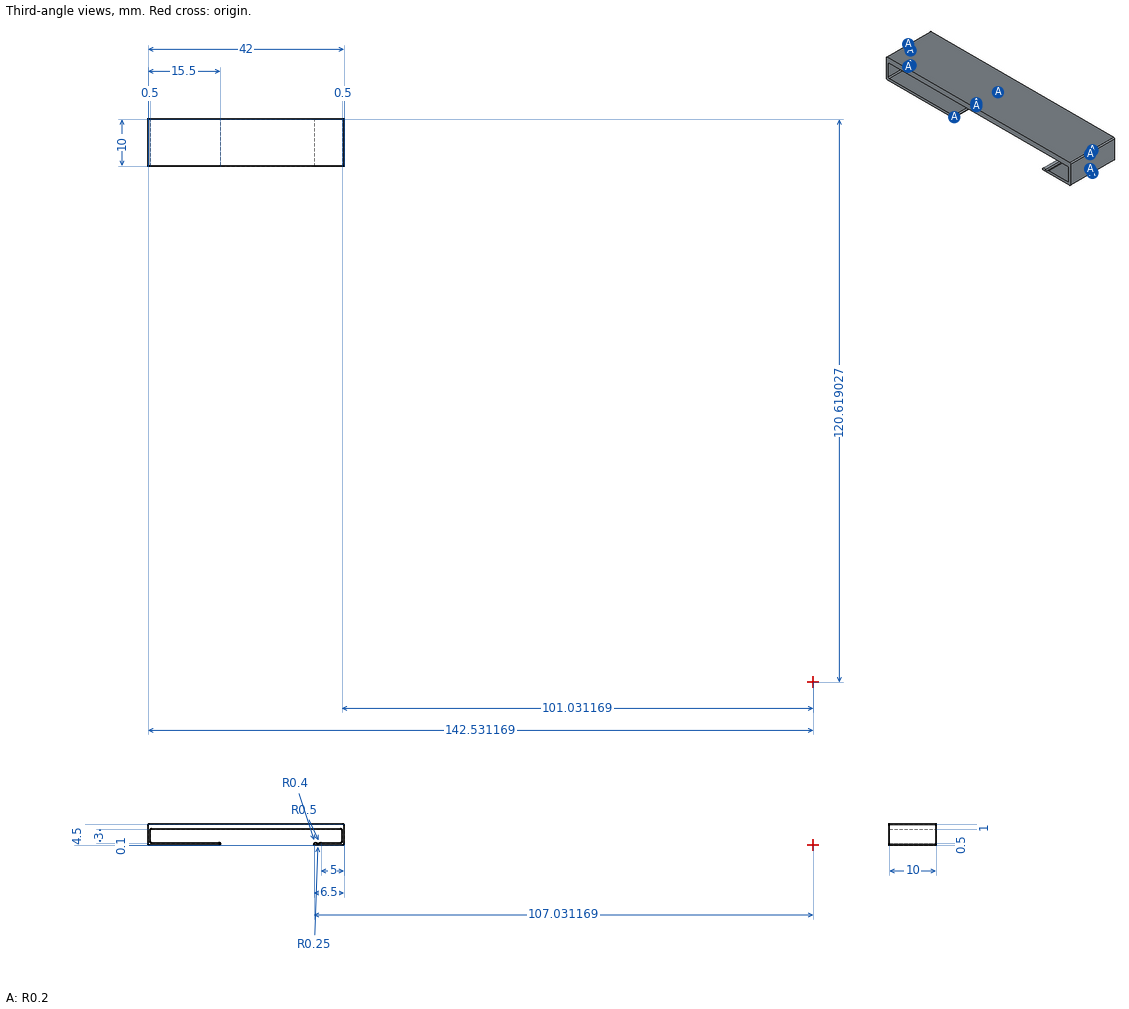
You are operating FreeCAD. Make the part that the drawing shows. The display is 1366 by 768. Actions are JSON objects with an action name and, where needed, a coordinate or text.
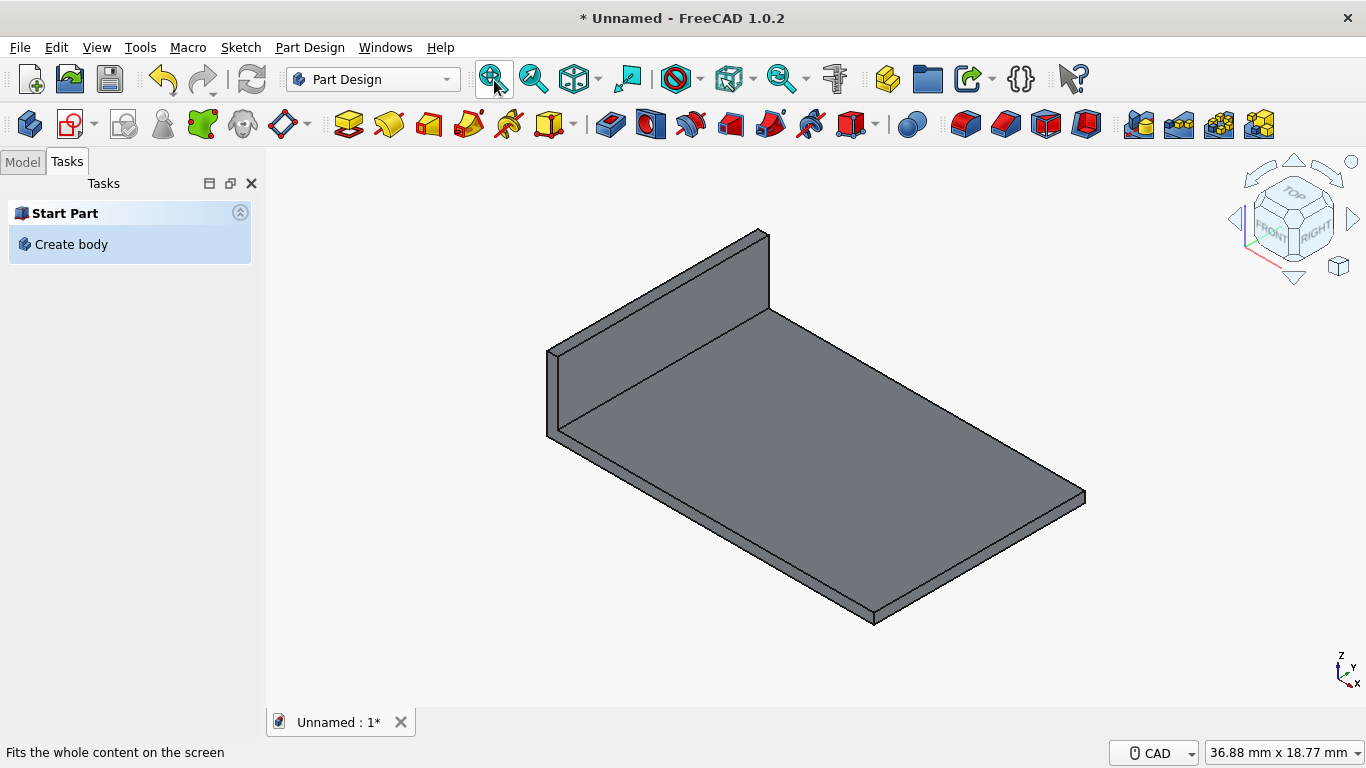
{"action": "key", "text": "2"}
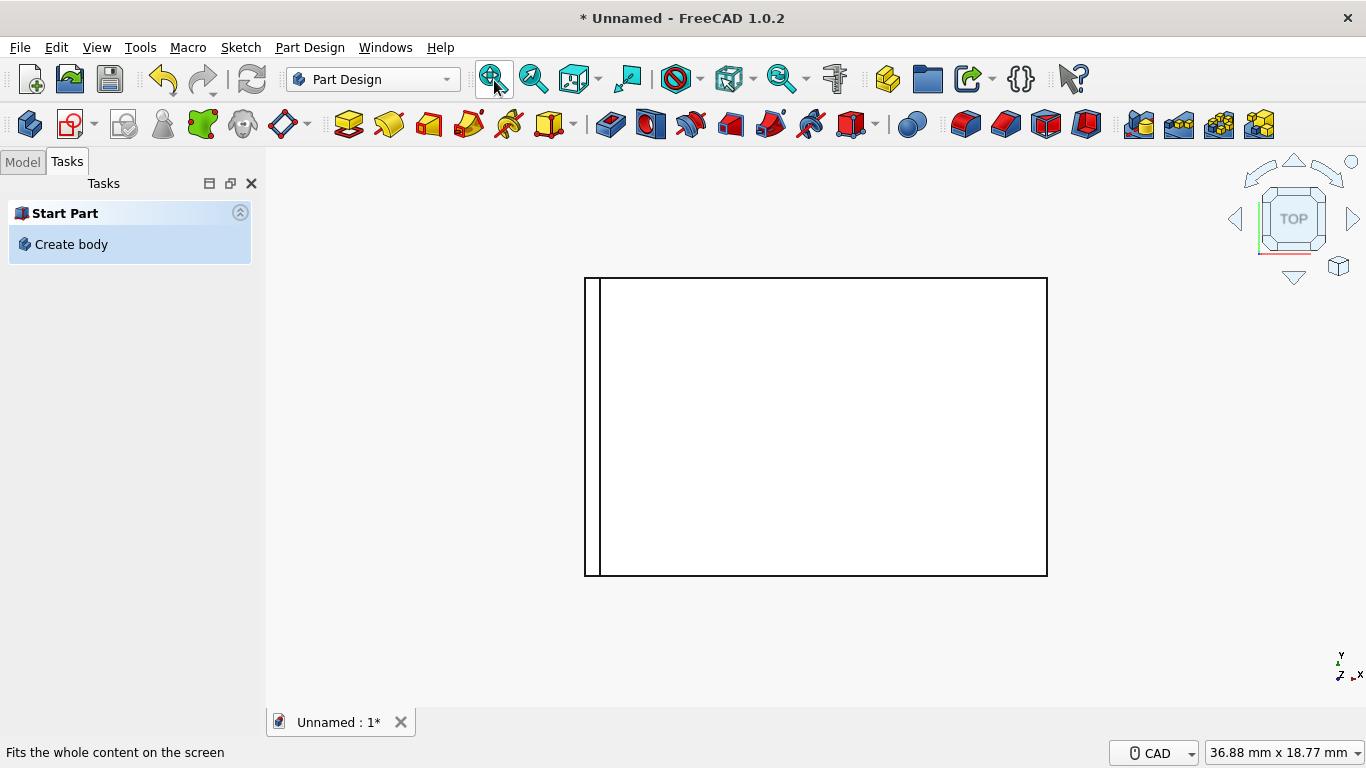
{"action": "key", "text": "1"}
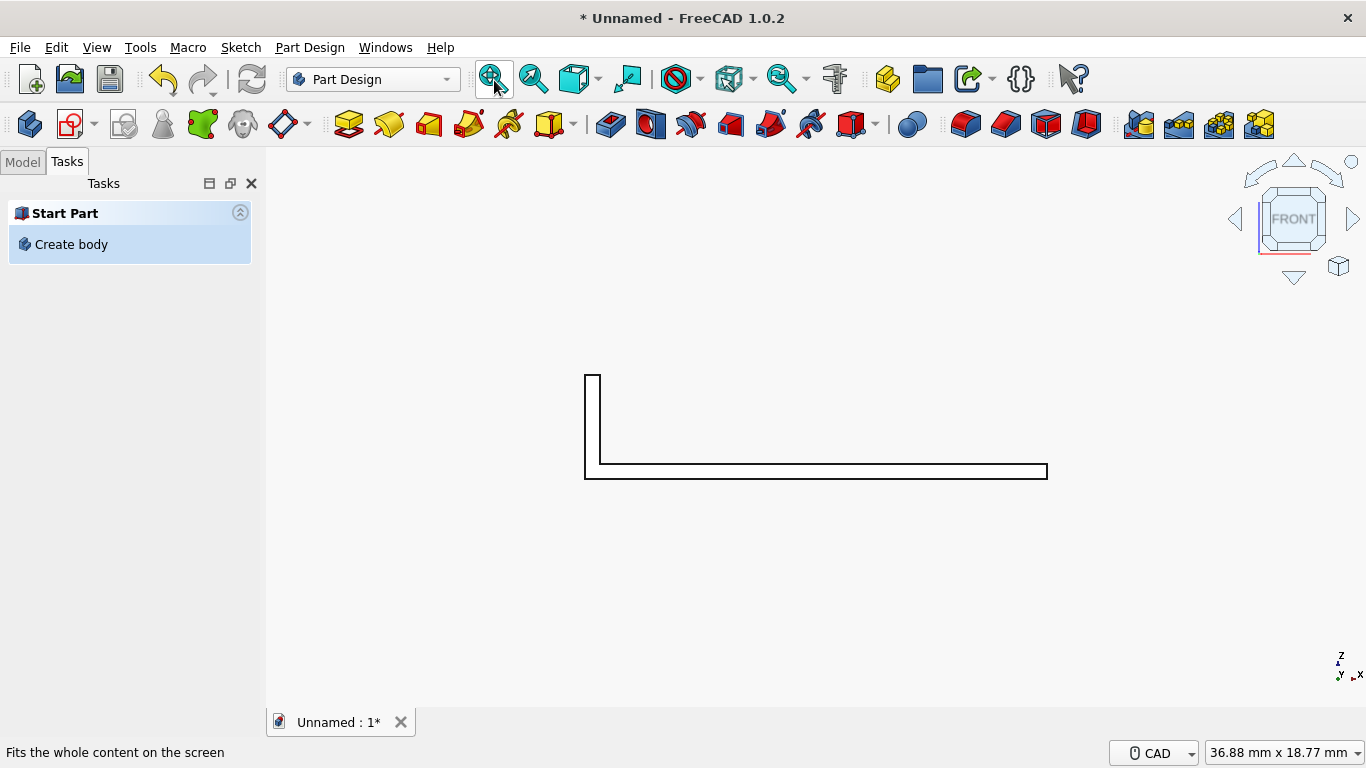
{"action": "left_click", "coordinate": [494, 80]}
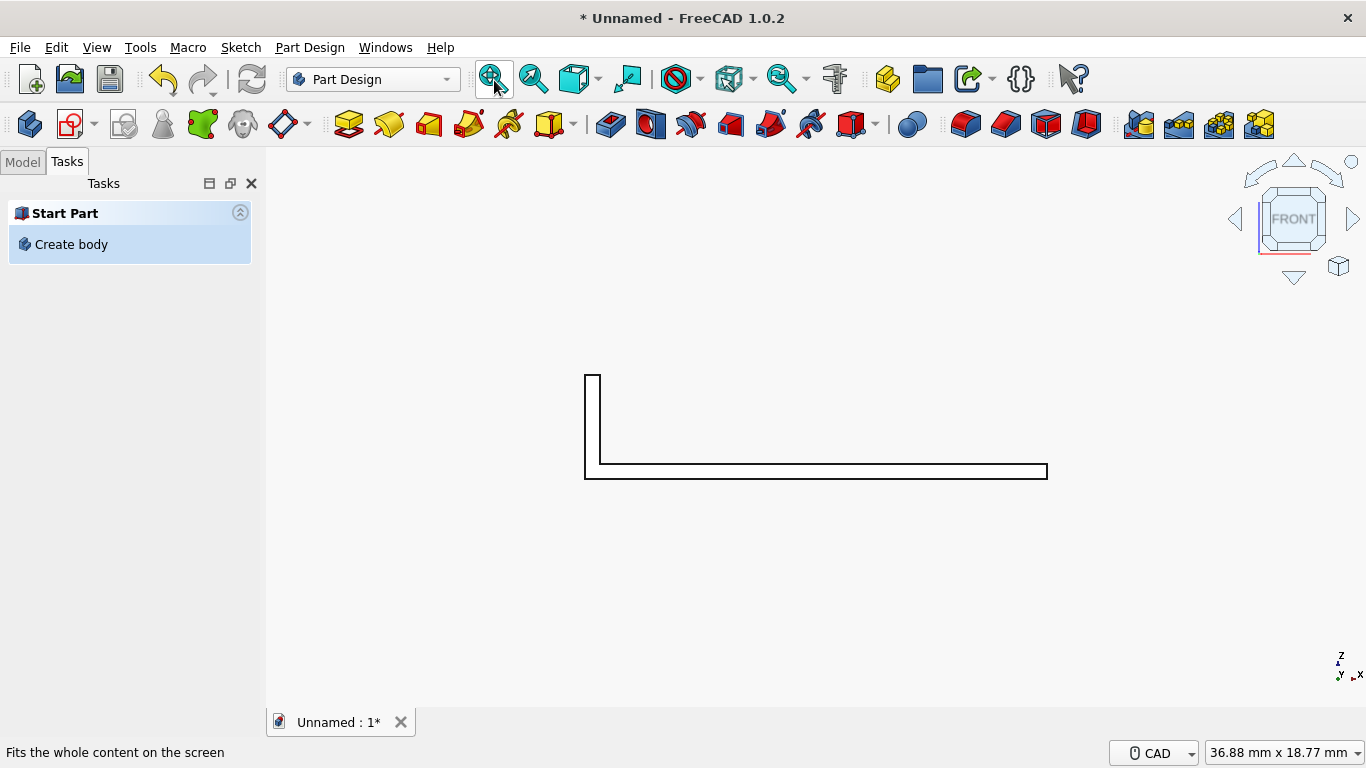
{"action": "left_click", "coordinate": [23, 161]}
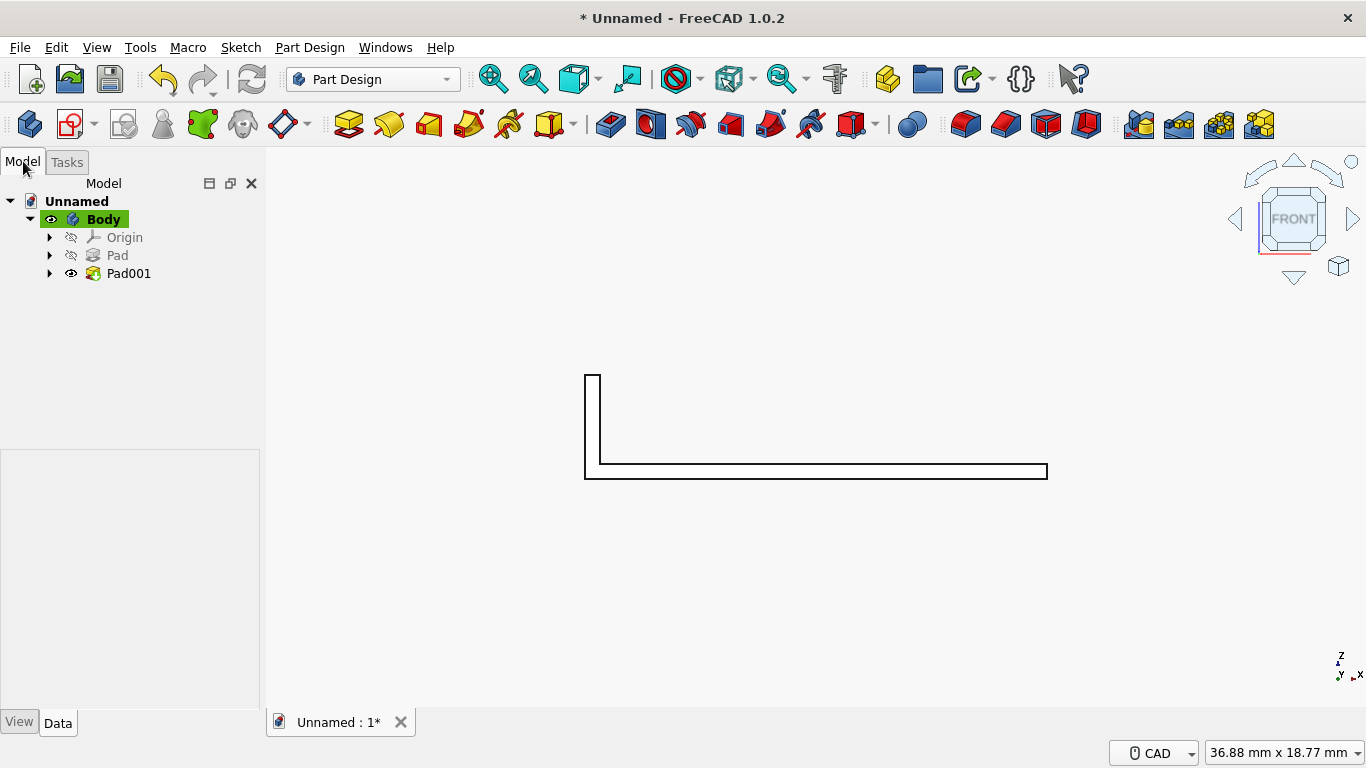
{"action": "left_click", "coordinate": [50, 237]}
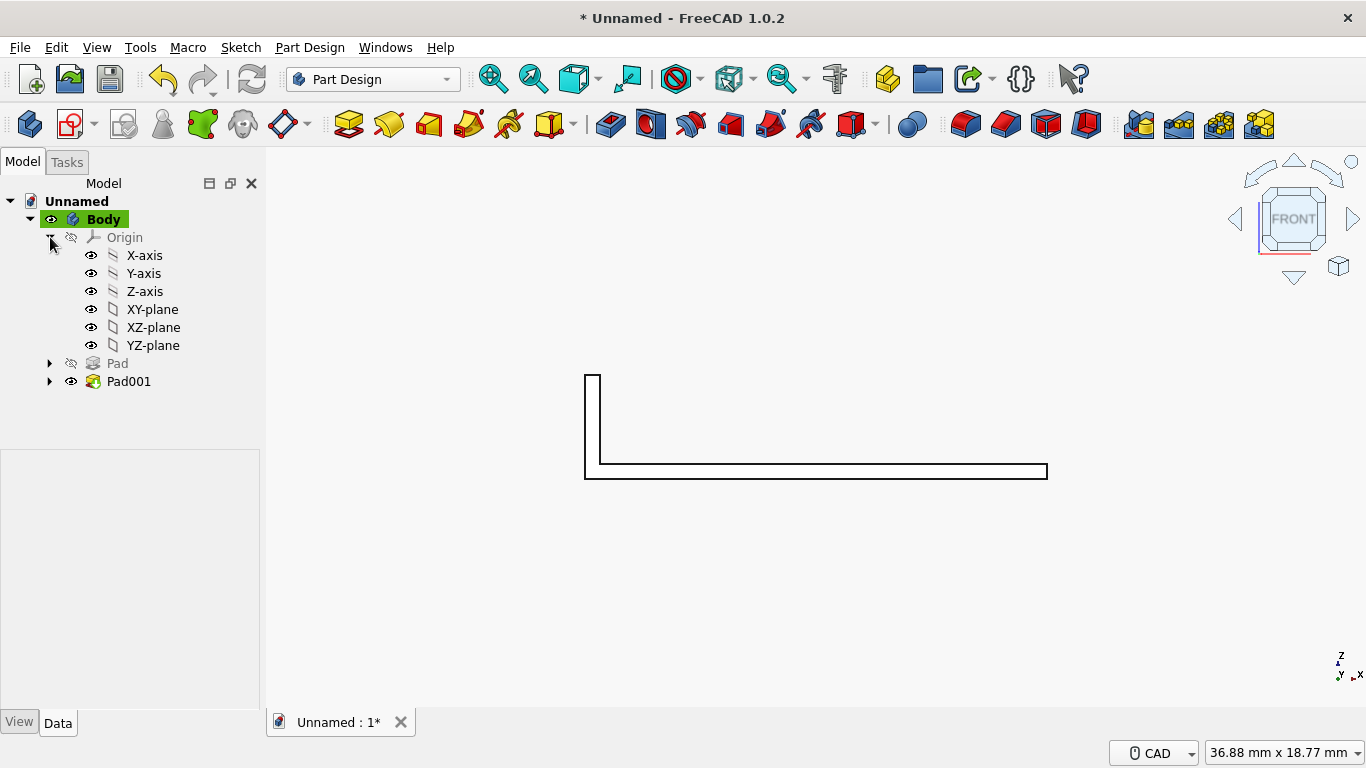
{"action": "left_click", "coordinate": [136, 309]}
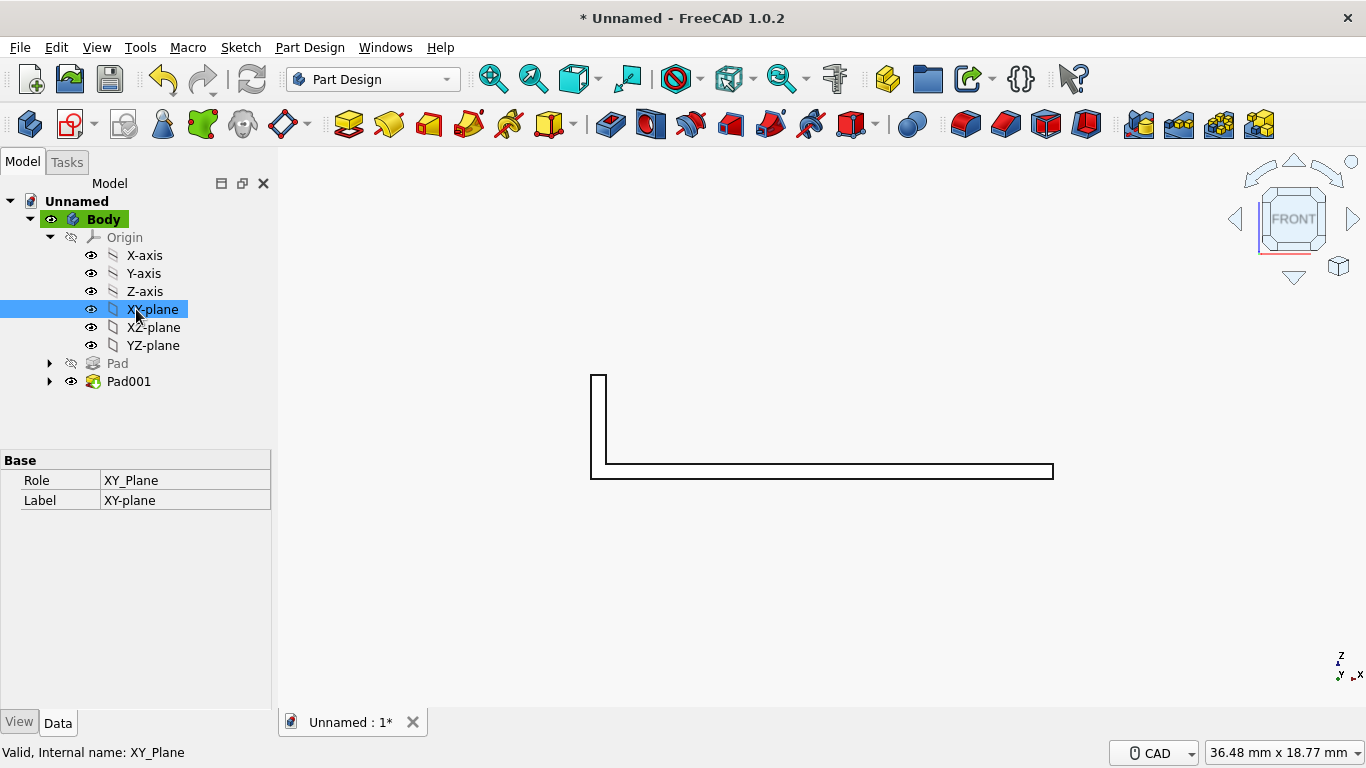
{"action": "left_click", "coordinate": [284, 124]}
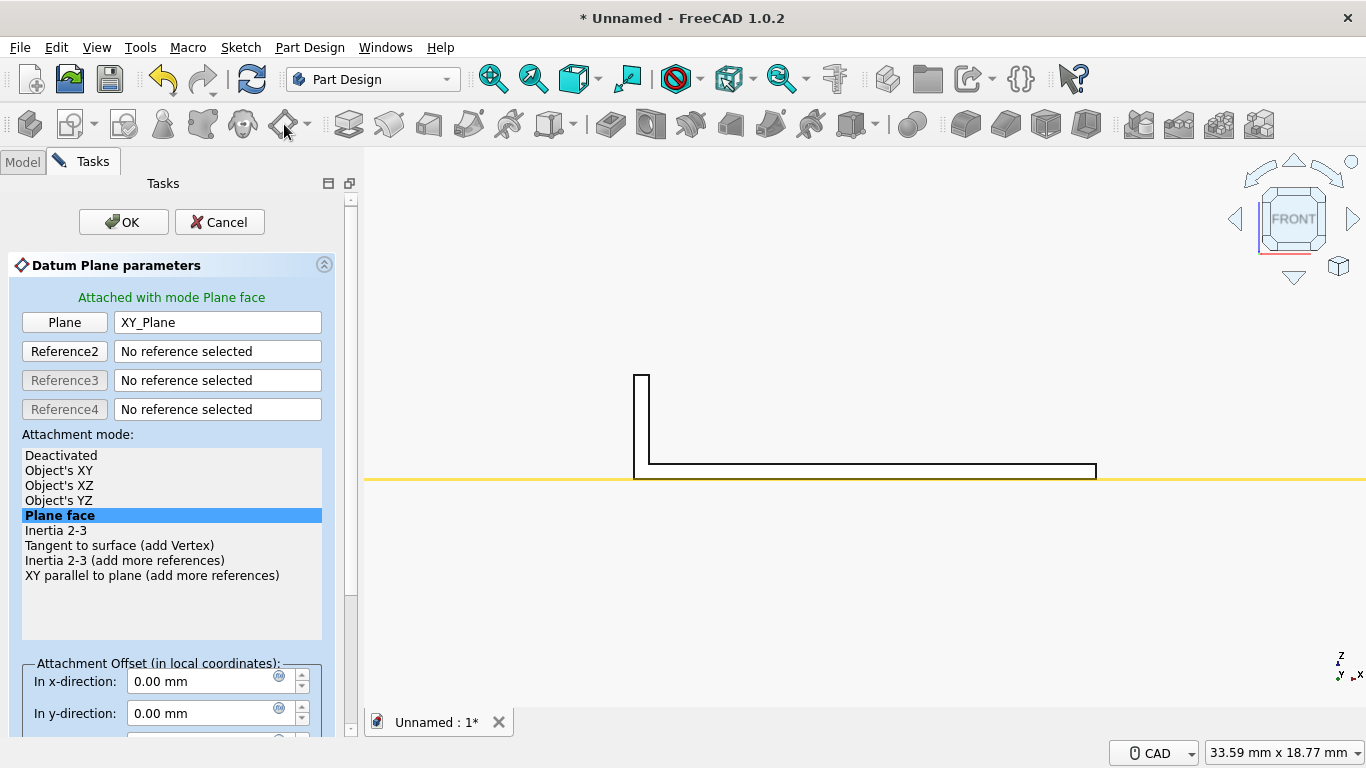
{"action": "scroll", "coordinate": [351, 464], "scroll_direction": "down", "scroll_amount": 2}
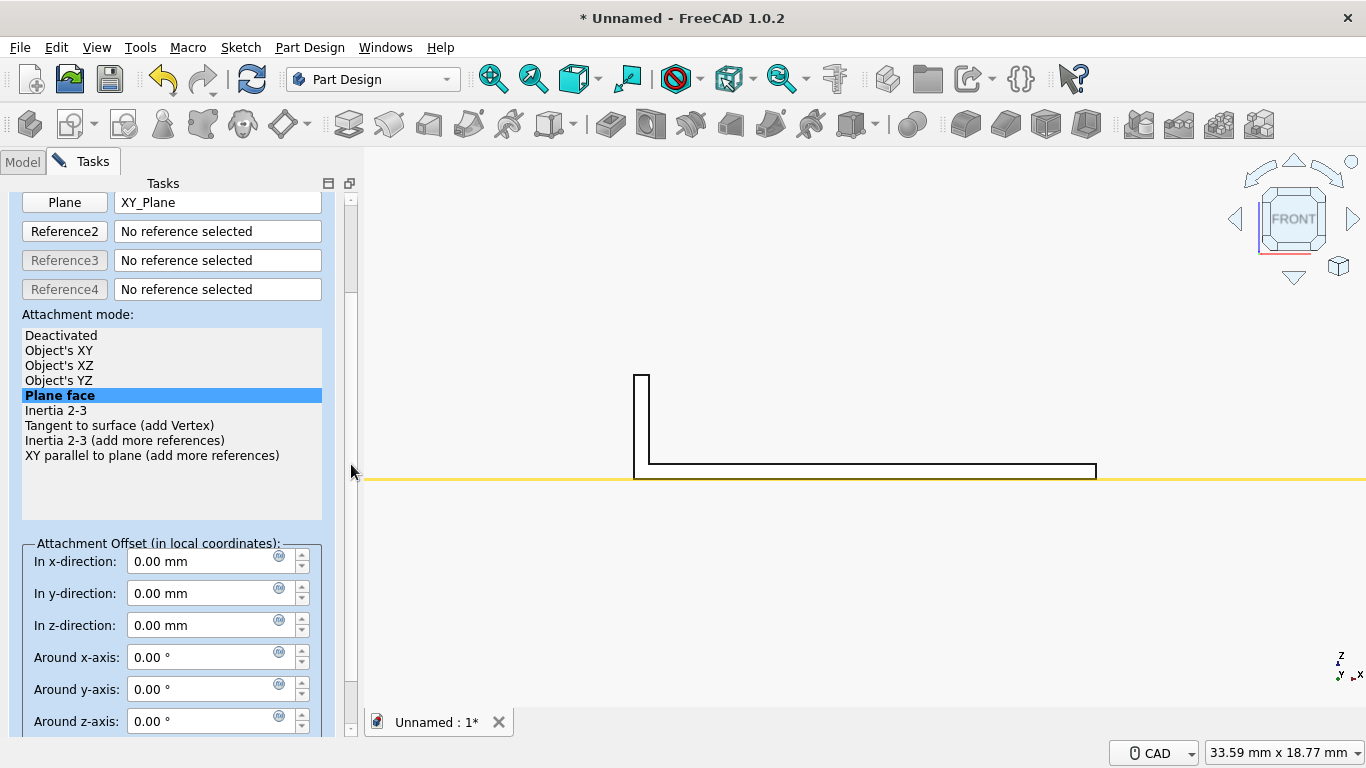
{"action": "triple_click", "coordinate": [210, 625]}